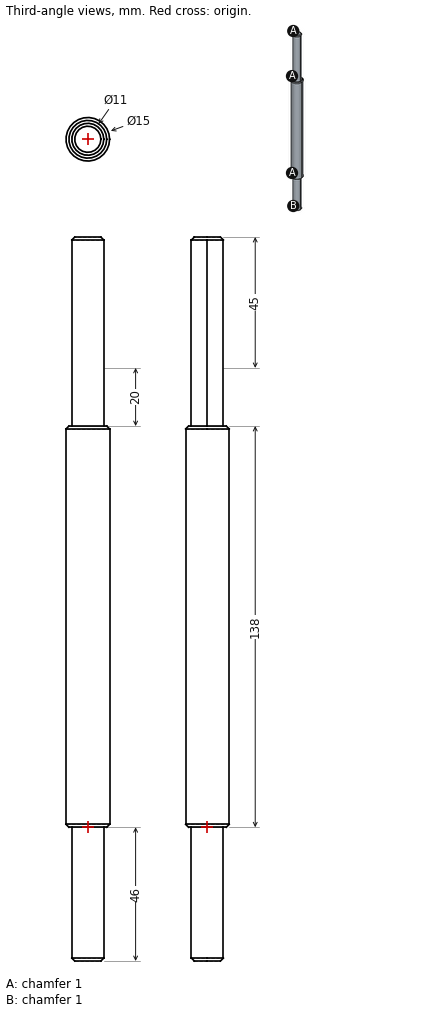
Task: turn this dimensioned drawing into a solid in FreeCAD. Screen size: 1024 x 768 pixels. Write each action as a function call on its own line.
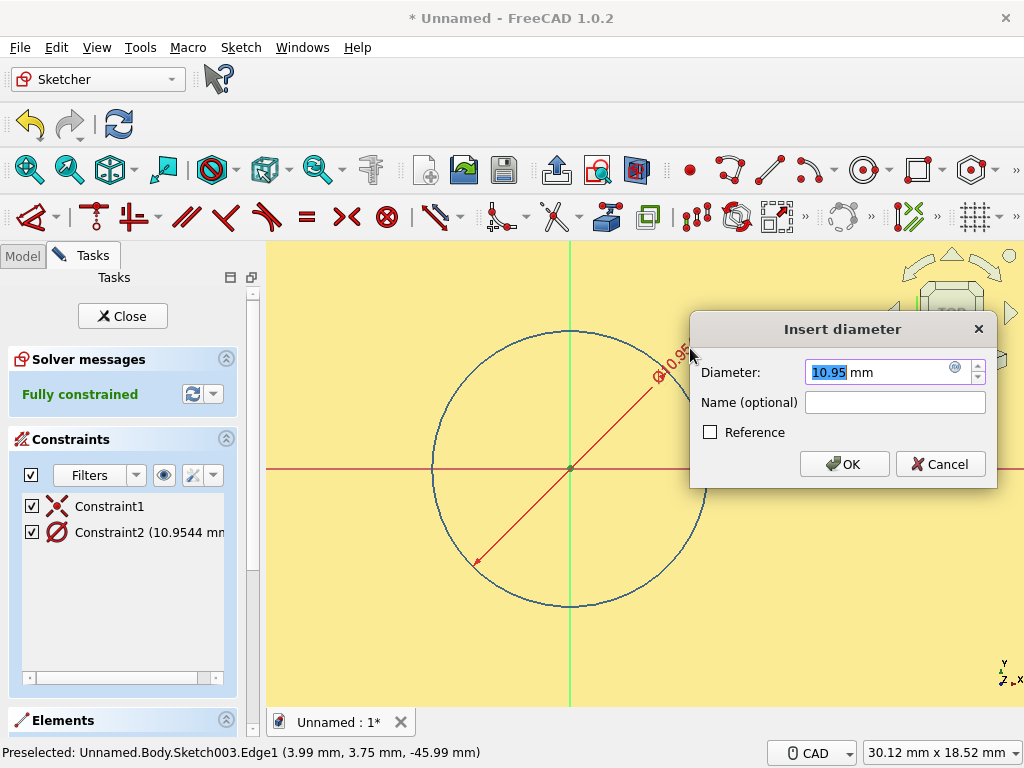
text(11)
key(Return)
key(Escape)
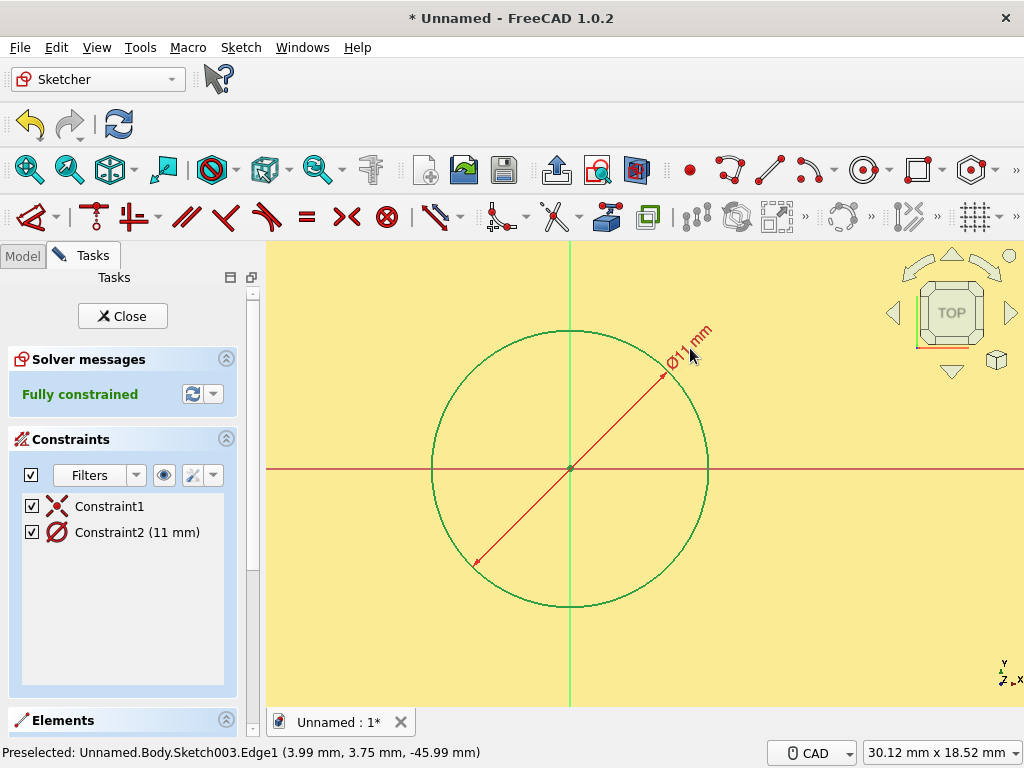
click(123, 316)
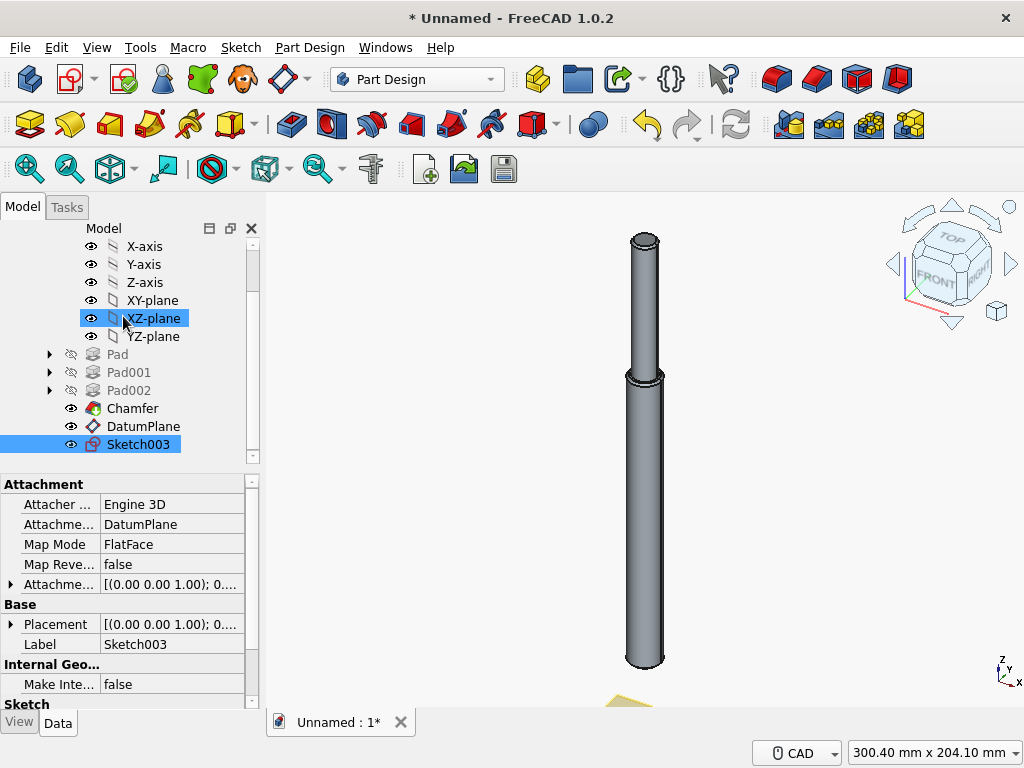
click(30, 124)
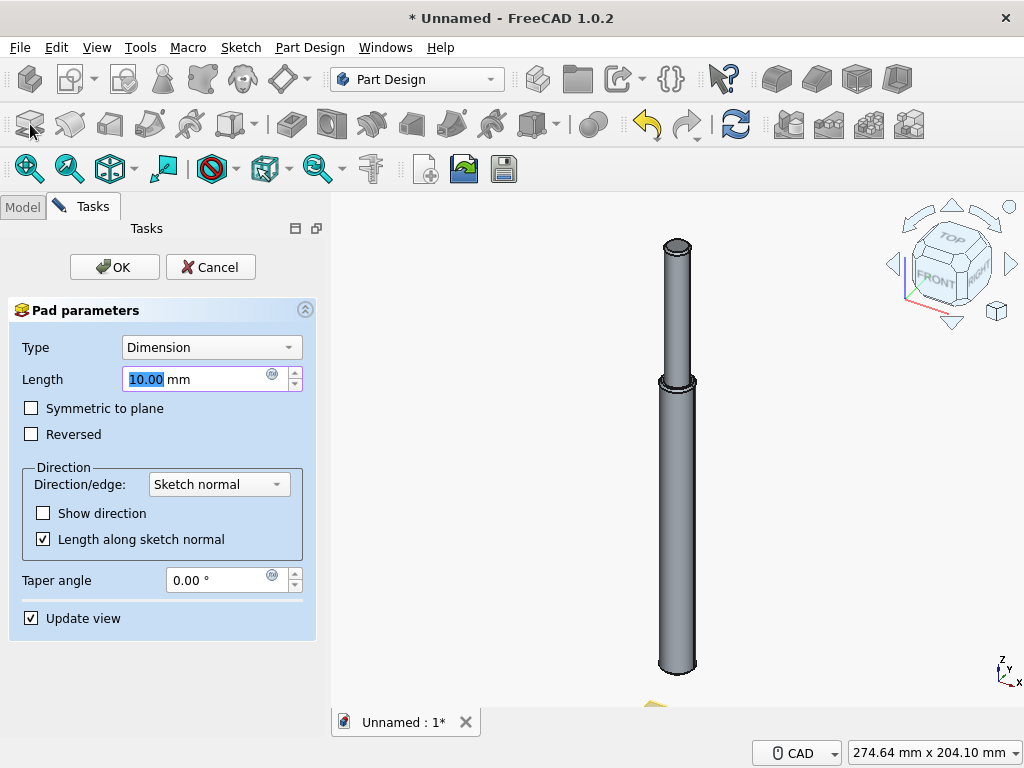
text(46)
key(Tab)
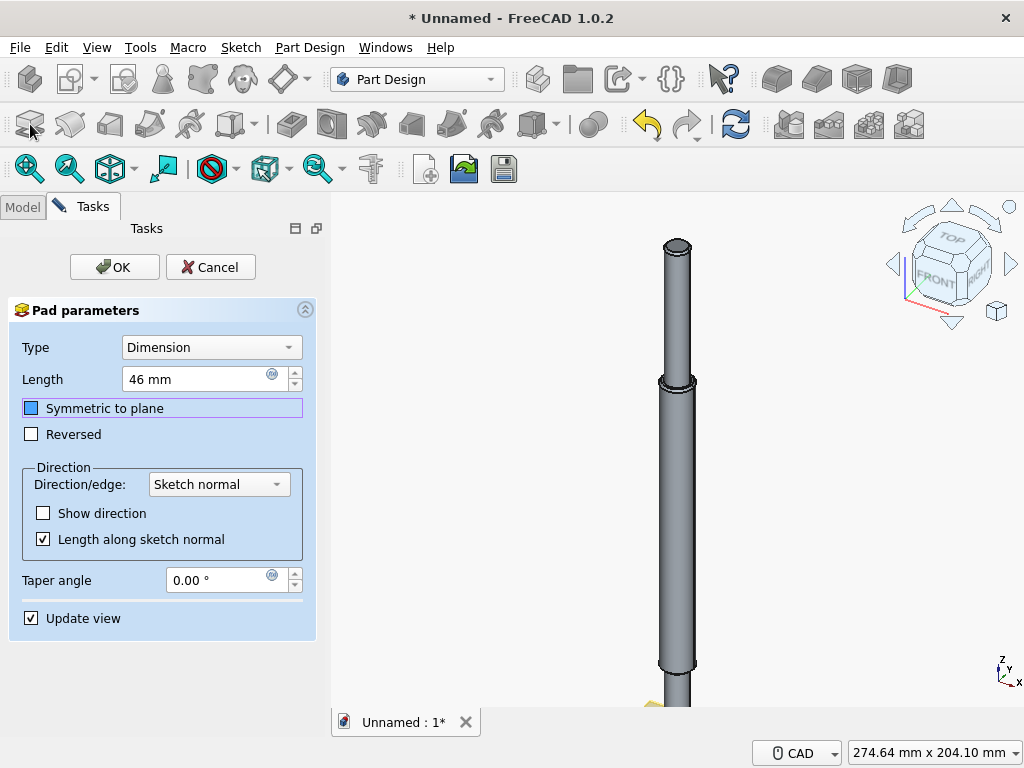
click(115, 267)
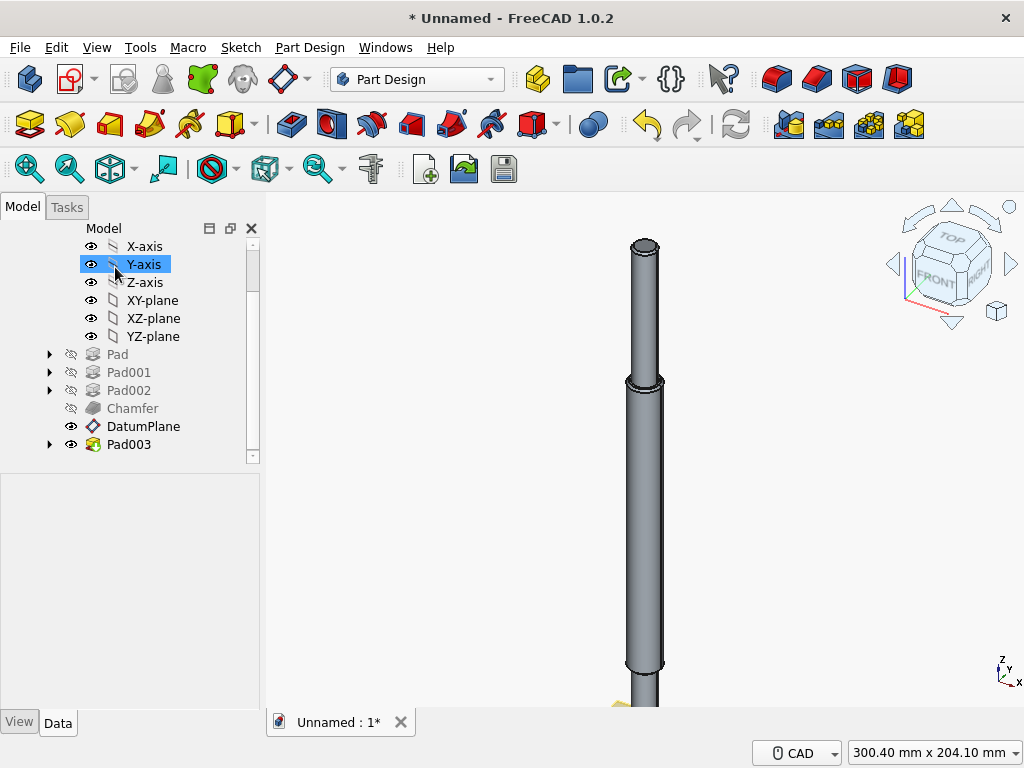
click(116, 426)
key(space)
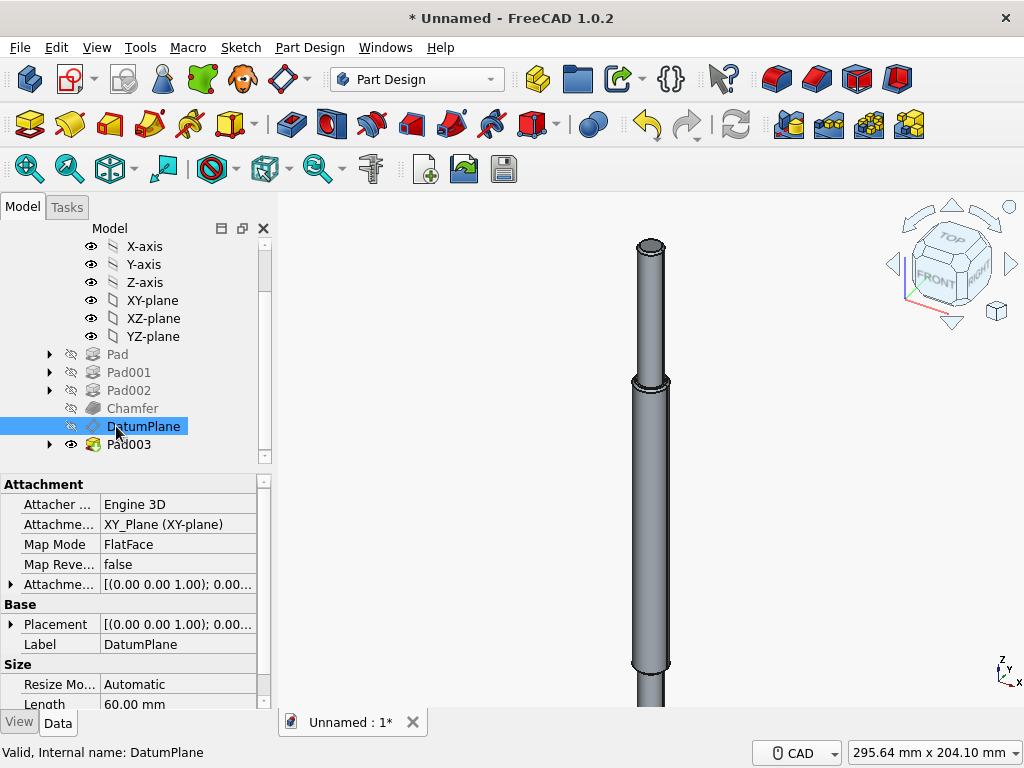
click(30, 170)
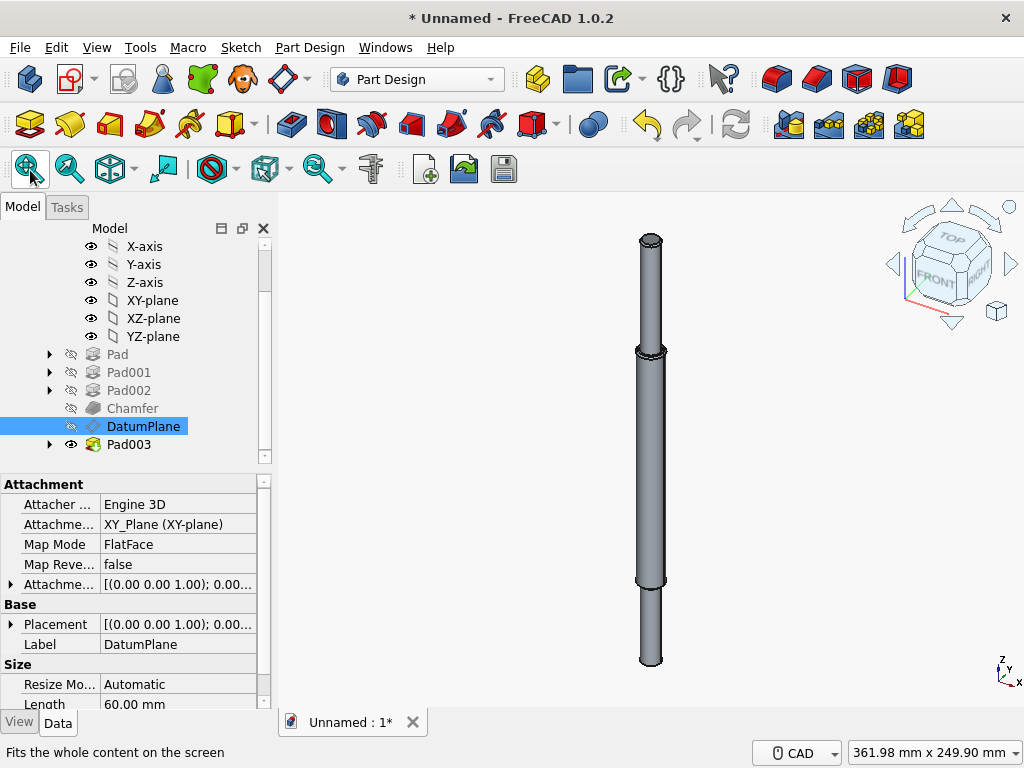
click(643, 663)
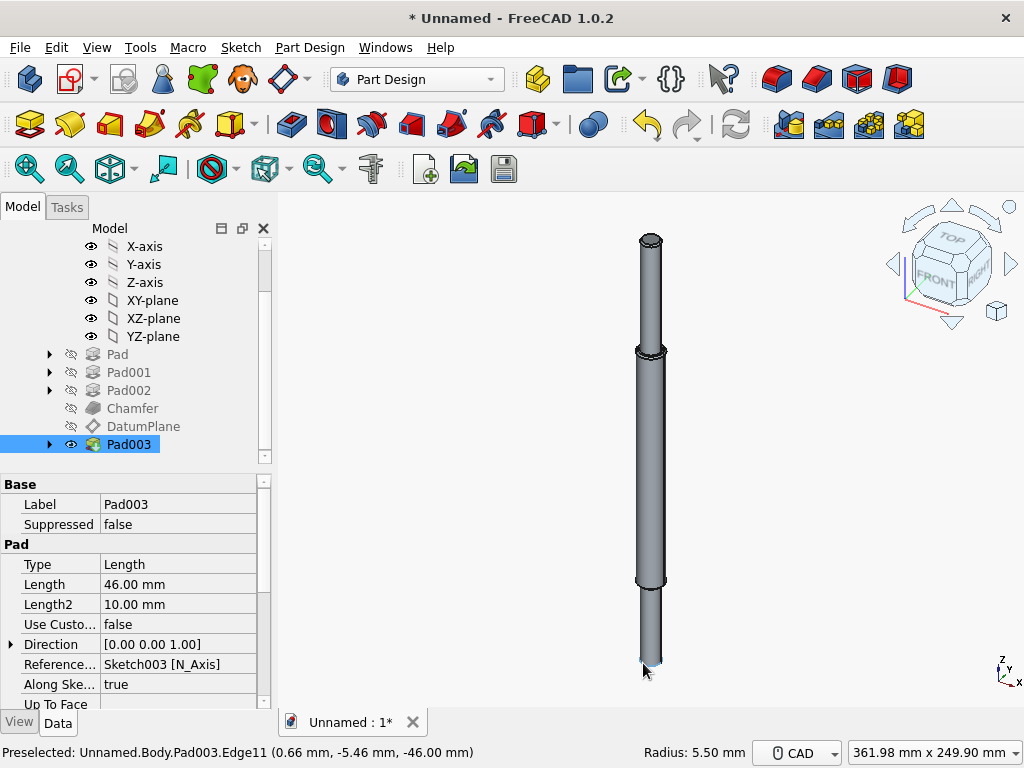
click(818, 80)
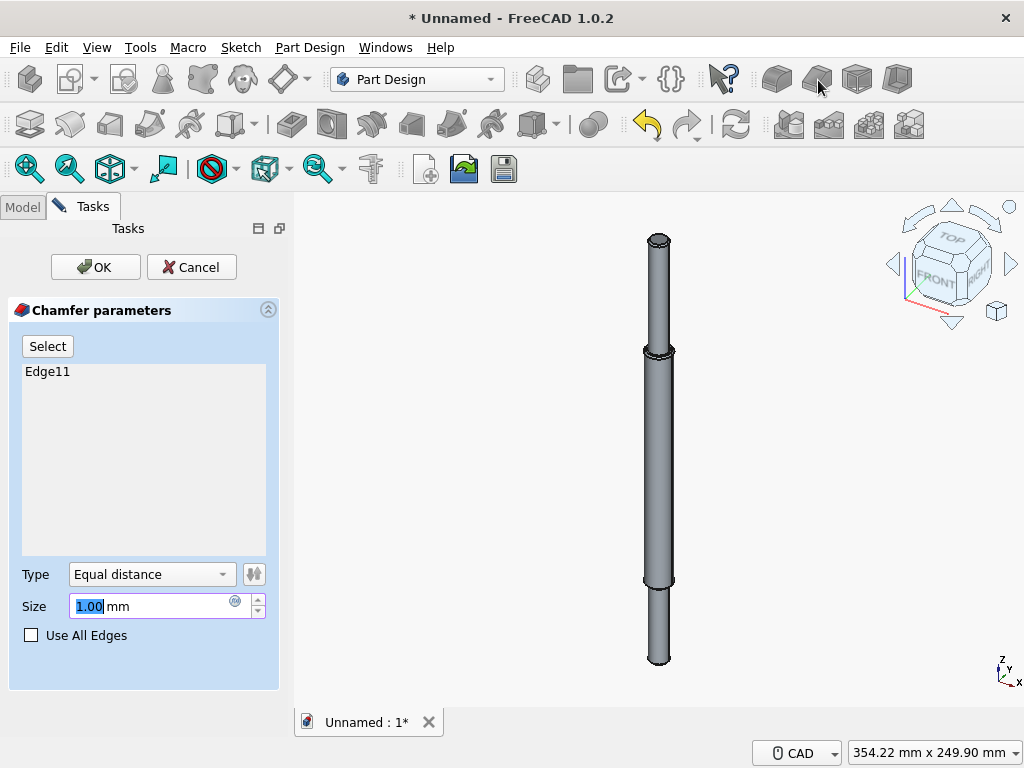
text(1)
key(Tab)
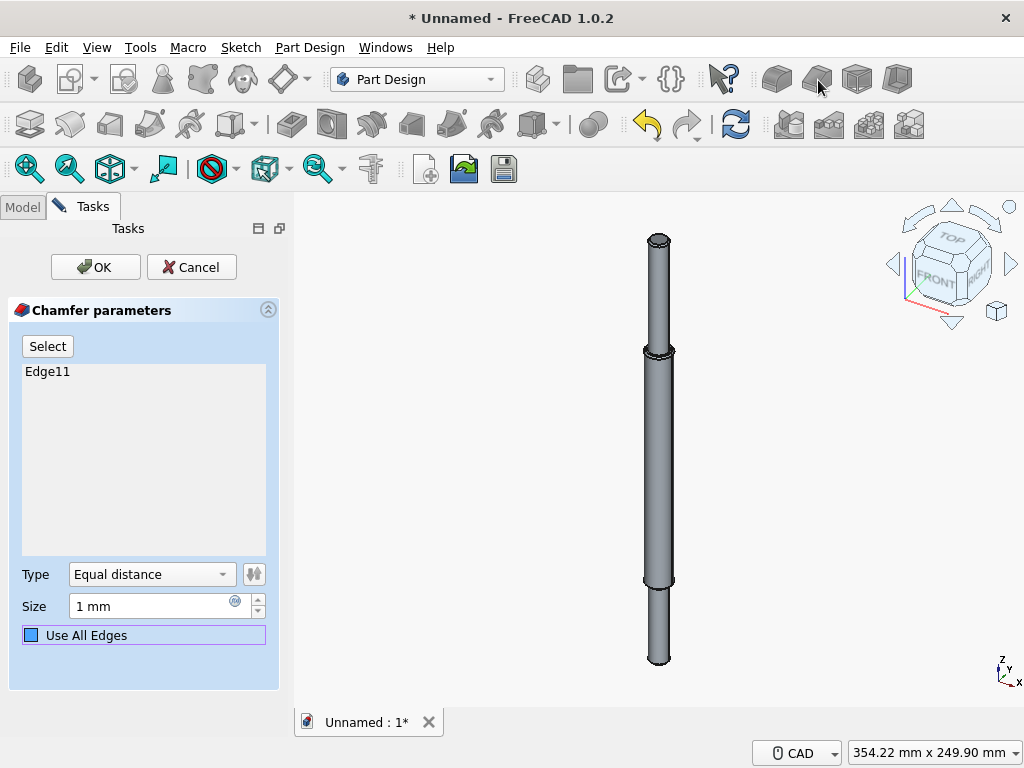
click(96, 267)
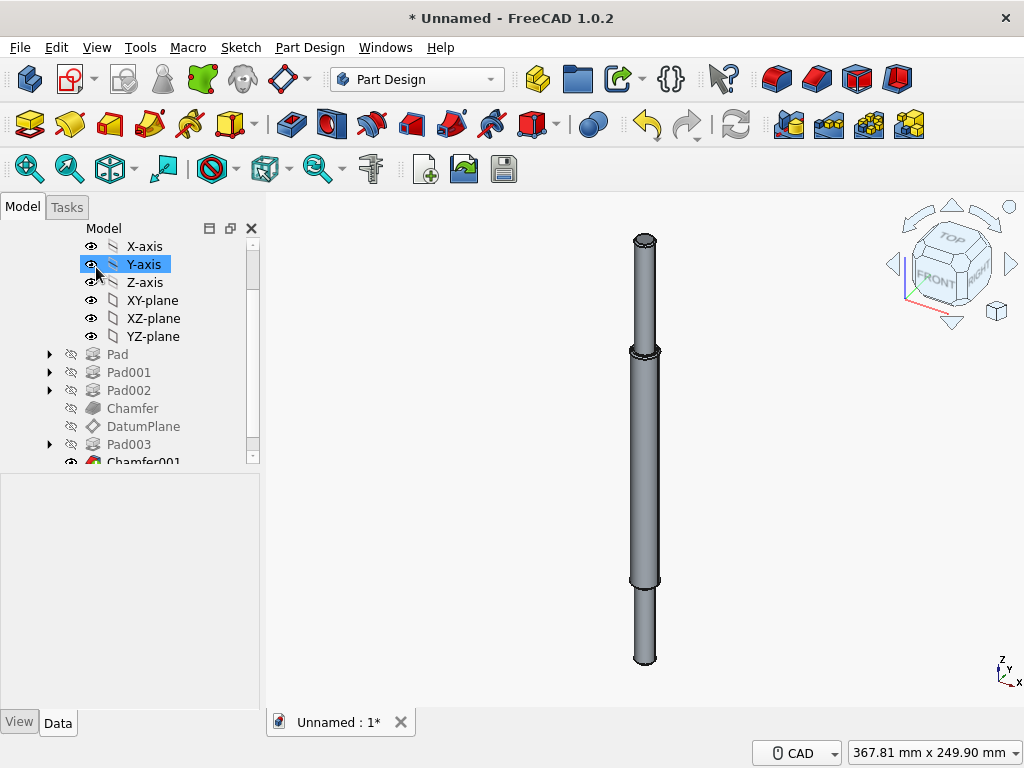
key(0)